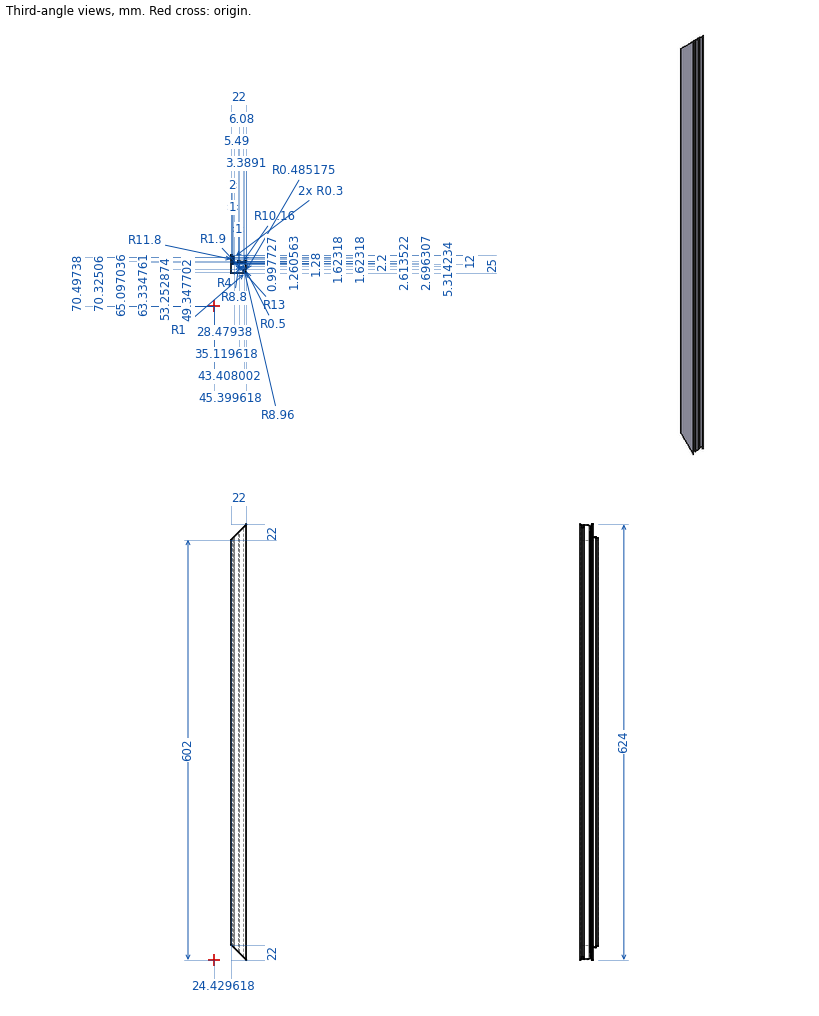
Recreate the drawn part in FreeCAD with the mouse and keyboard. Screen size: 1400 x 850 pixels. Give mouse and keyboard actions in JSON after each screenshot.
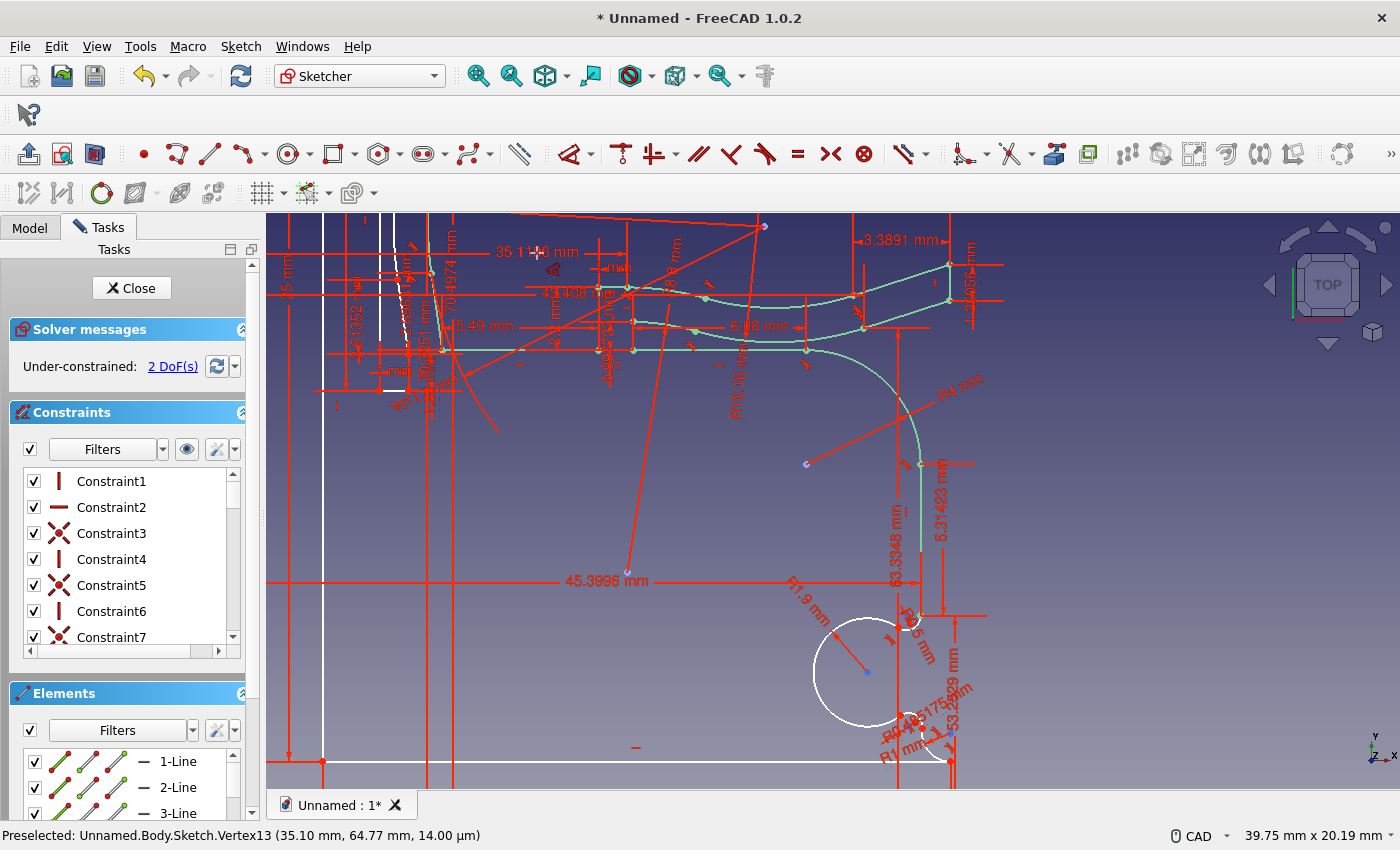
{"action": "left_click", "coordinate": [398, 280]}
{"action": "left_click", "coordinate": [432, 520]}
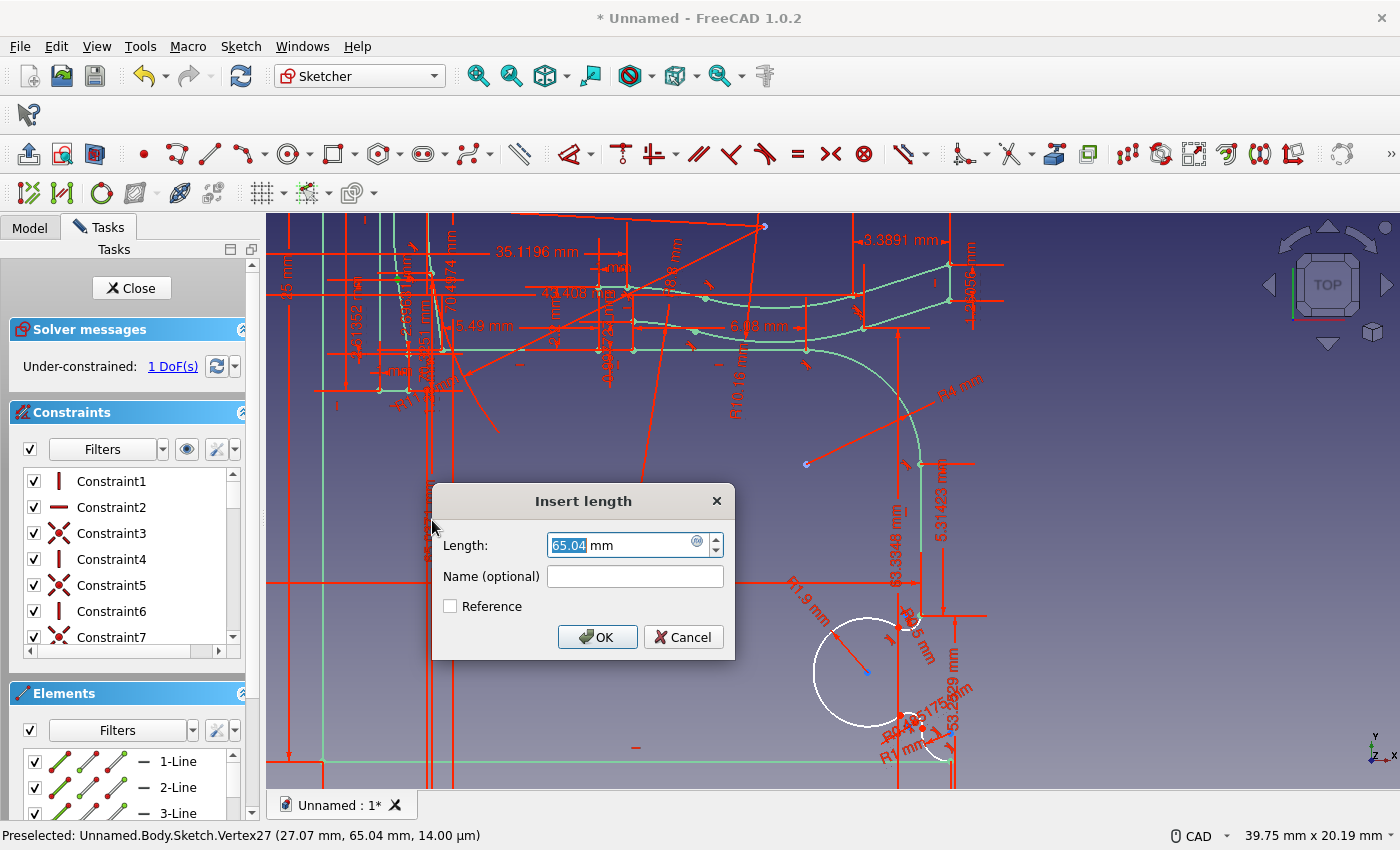
{"action": "type", "text": "65.097036"}
{"action": "key", "text": "Return"}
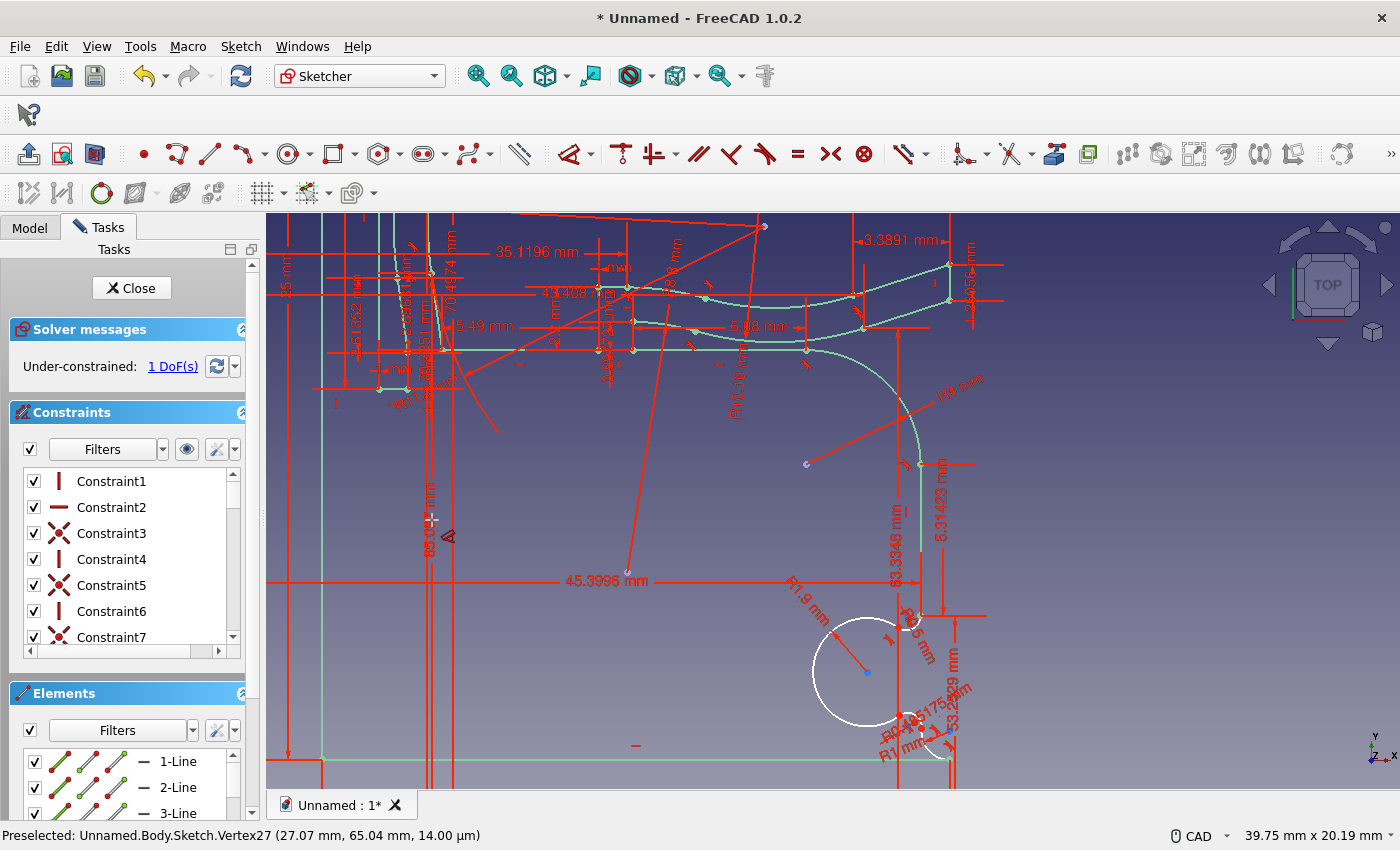
{"action": "left_click", "coordinate": [922, 728]}
{"action": "left_click", "coordinate": [980, 745]}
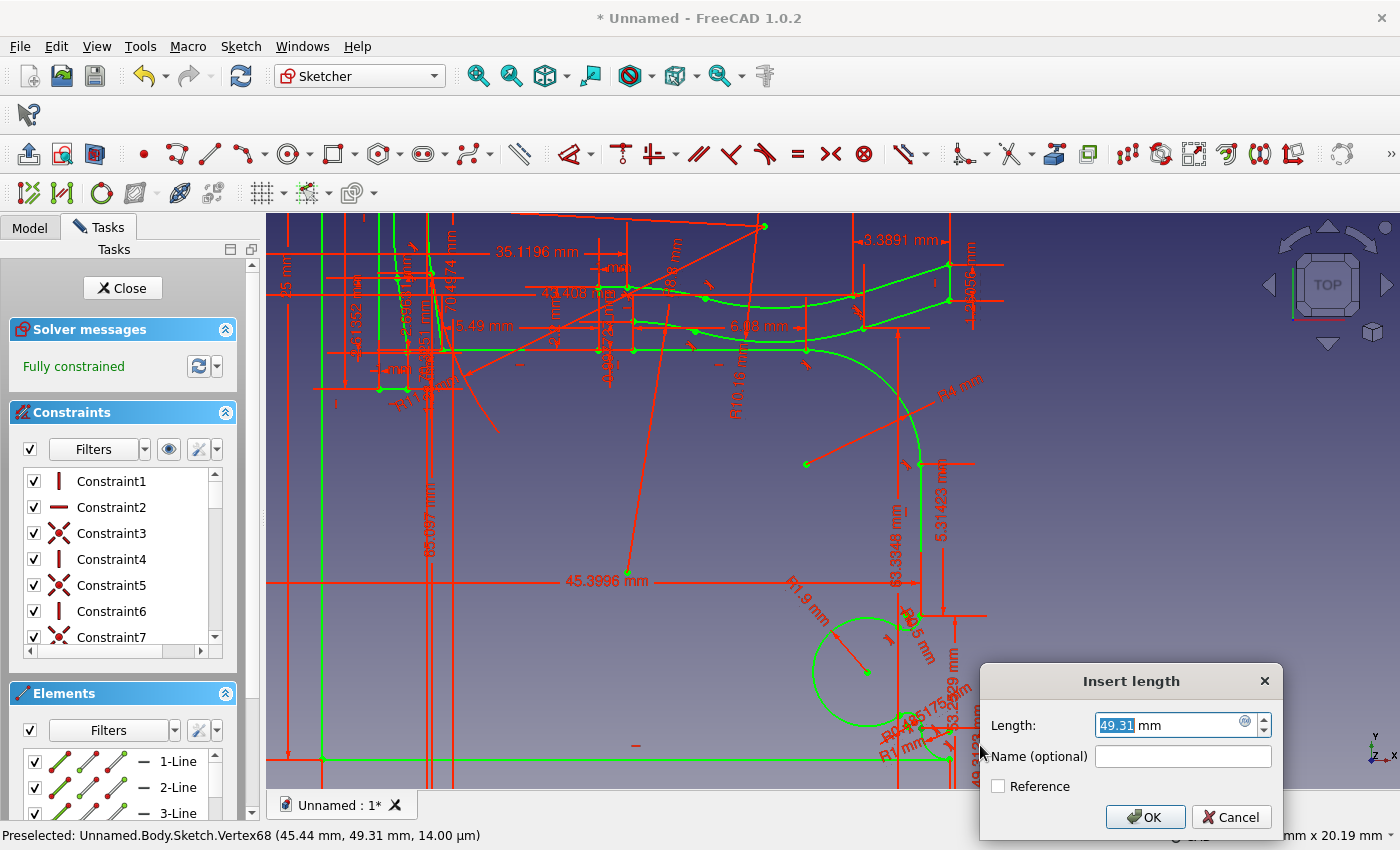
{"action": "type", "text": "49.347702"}
{"action": "key", "text": "Return"}
{"action": "key", "text": "Escape"}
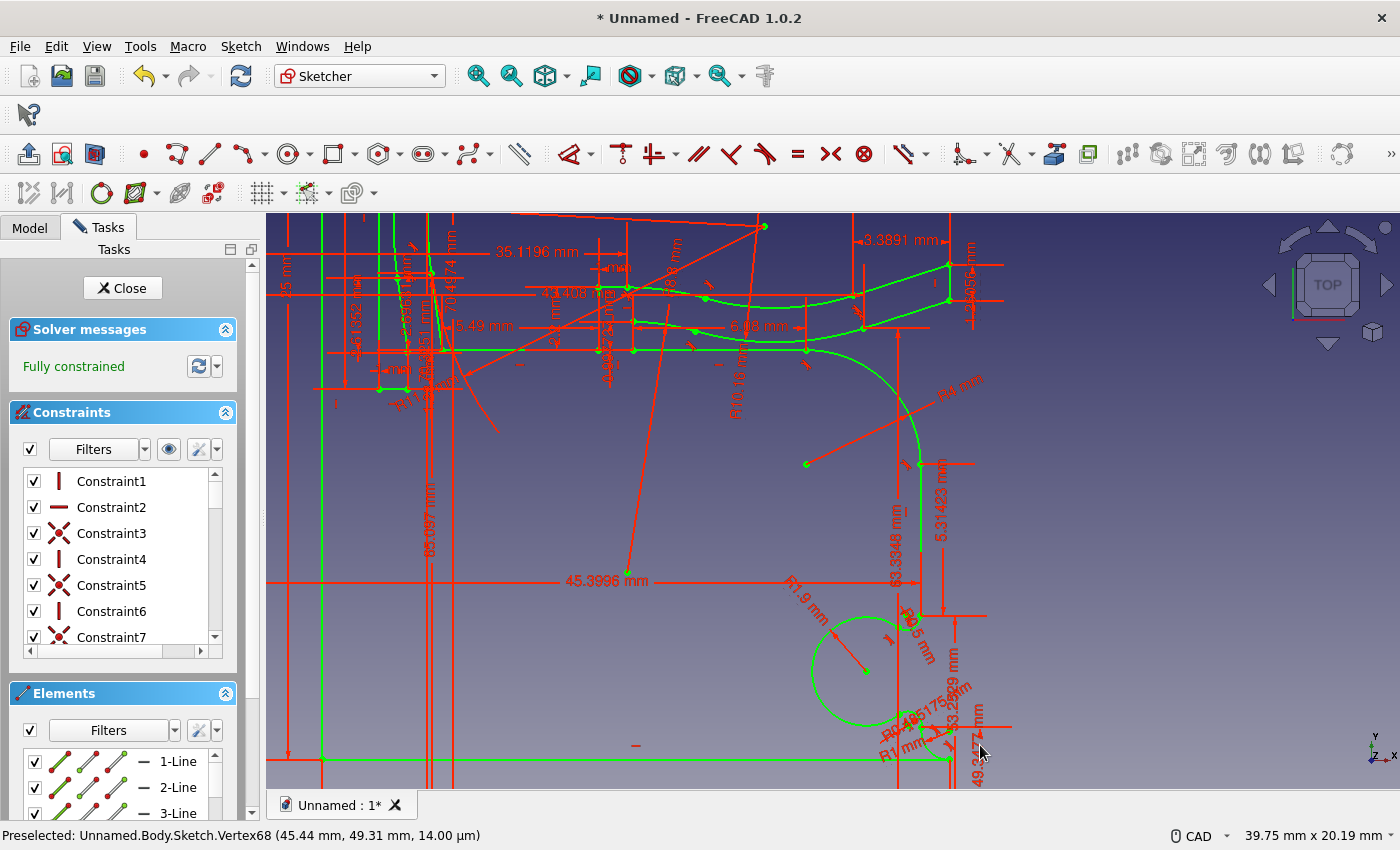
{"action": "left_click", "coordinate": [123, 288]}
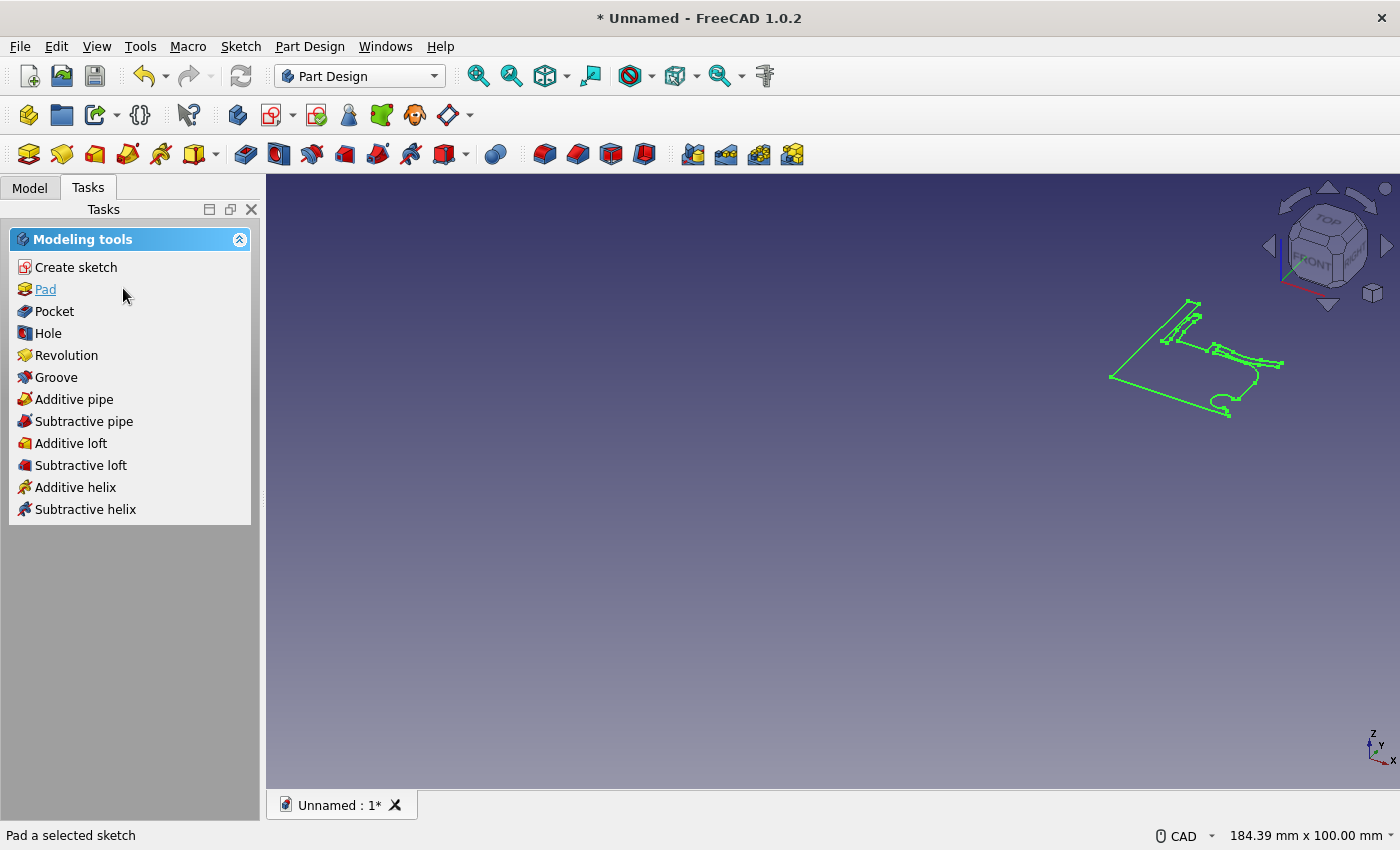
{"action": "left_click", "coordinate": [29, 154]}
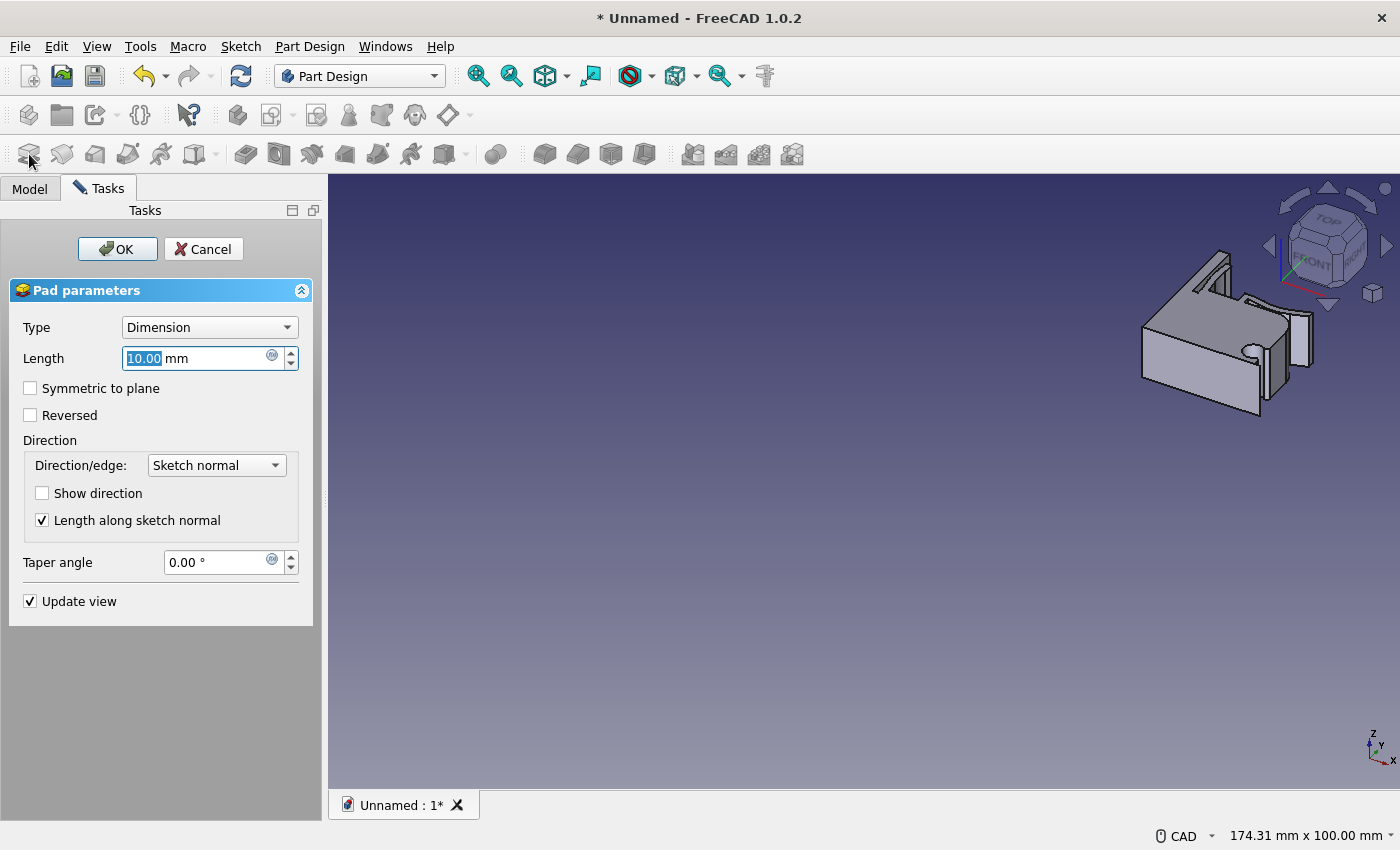
{"action": "type", "text": "624"}
{"action": "key", "text": "Tab"}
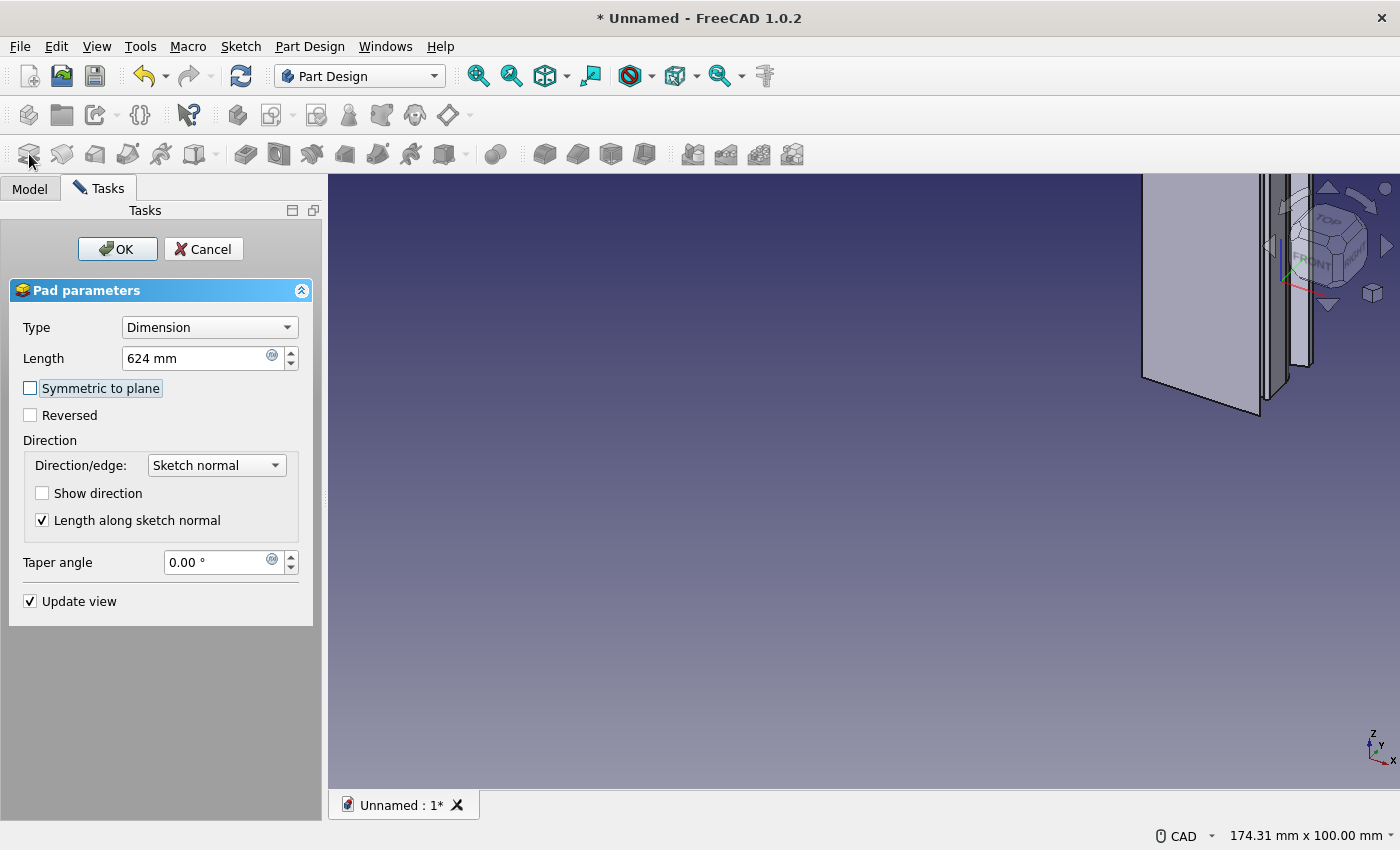
{"action": "left_click", "coordinate": [118, 249]}